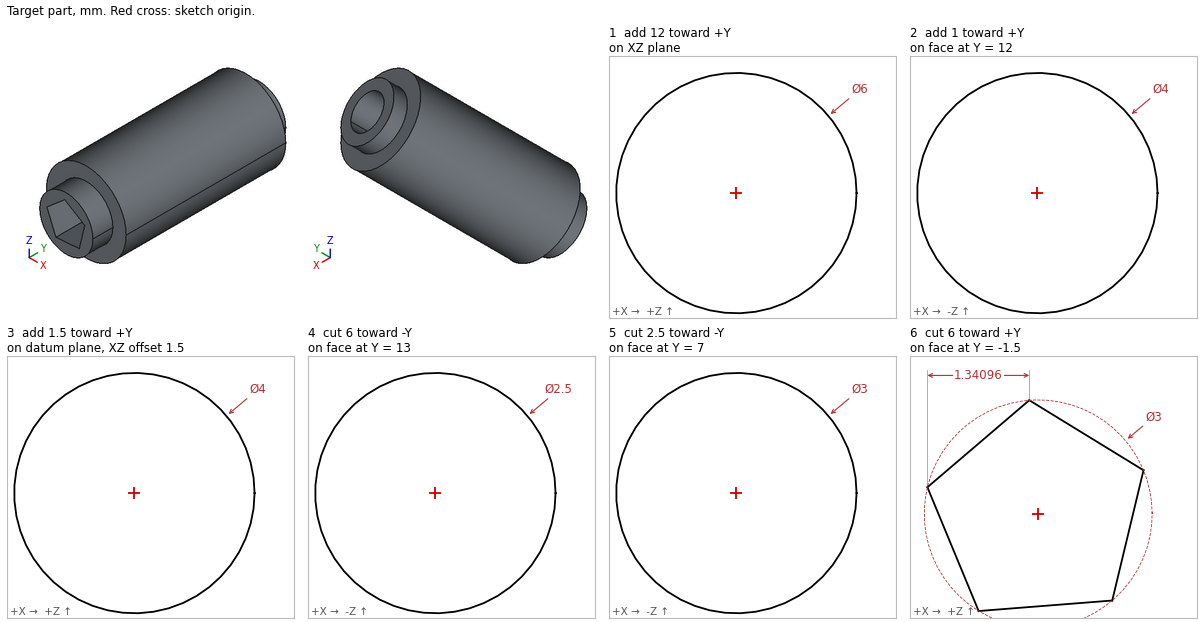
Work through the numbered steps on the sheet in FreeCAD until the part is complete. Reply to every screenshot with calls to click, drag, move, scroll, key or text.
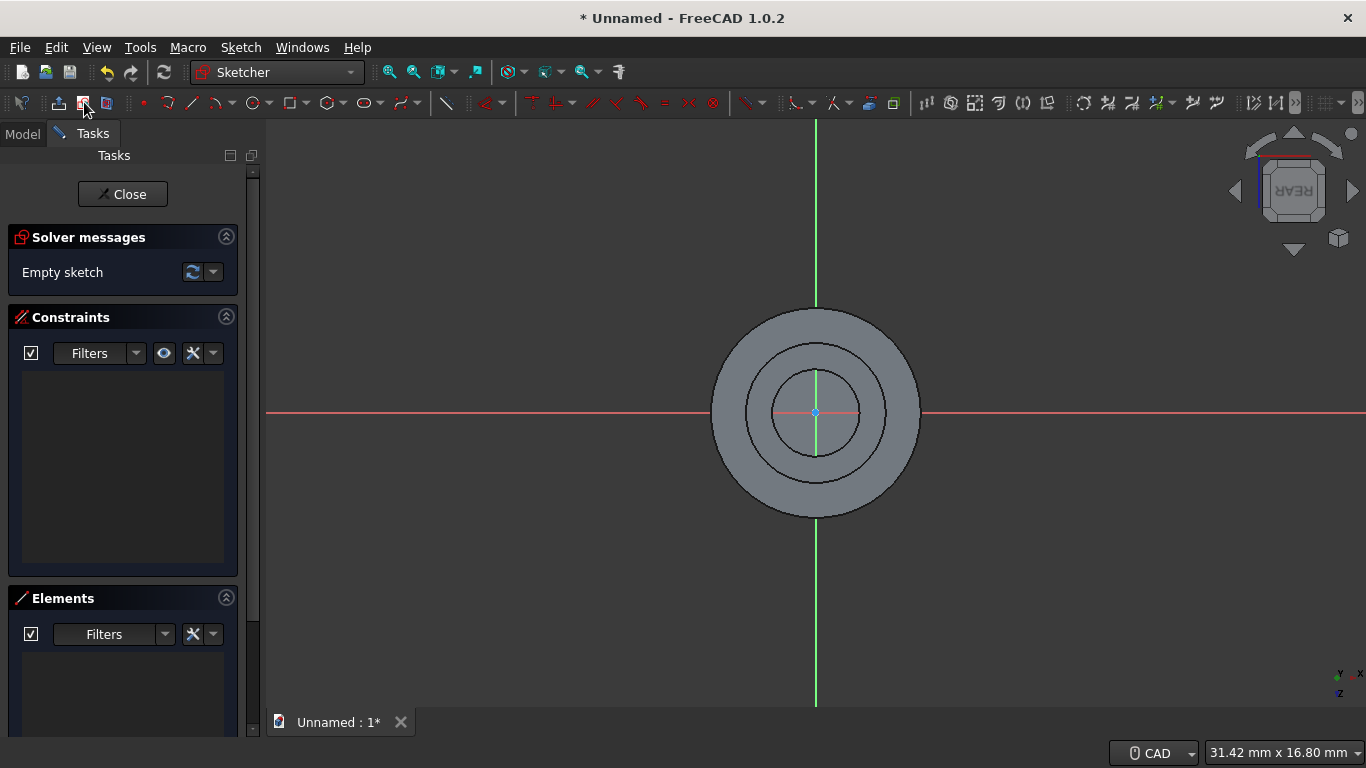
click(108, 104)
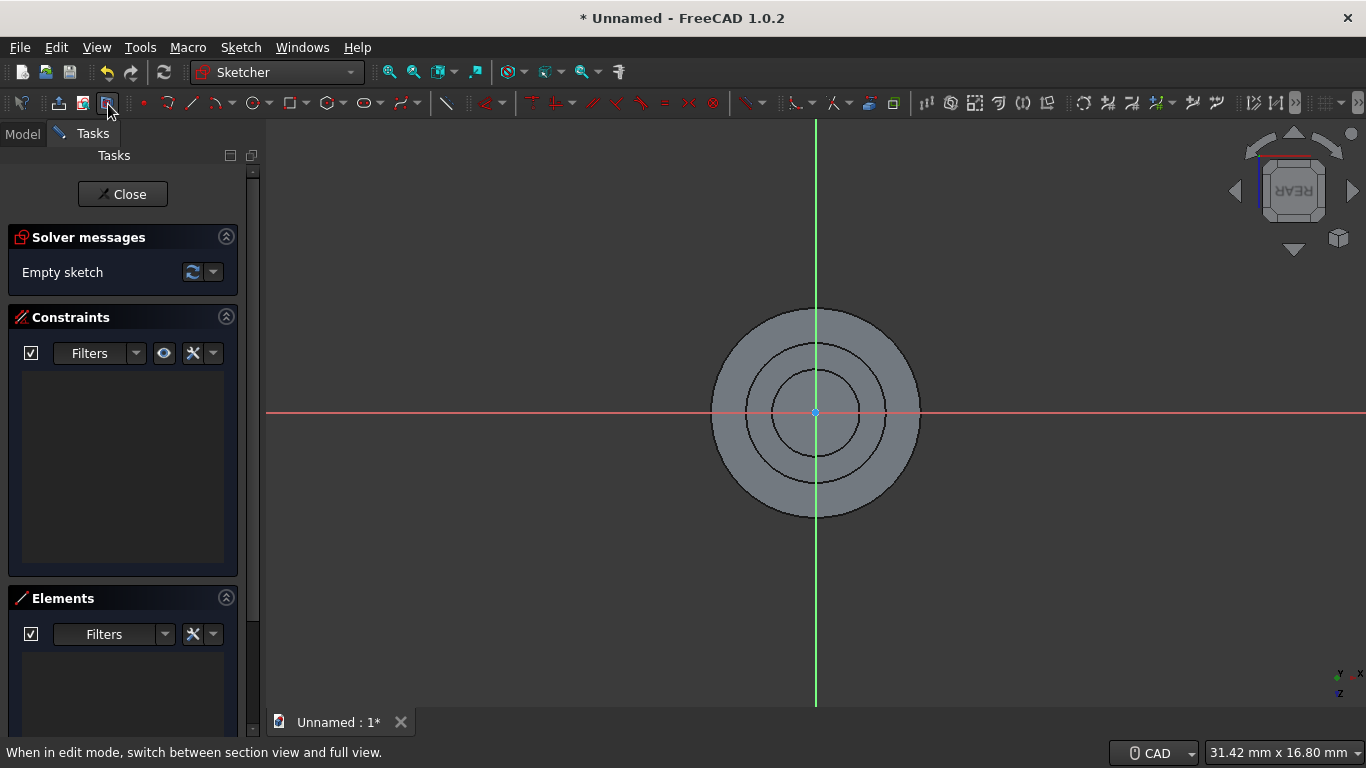
scroll(845, 413, up, 6)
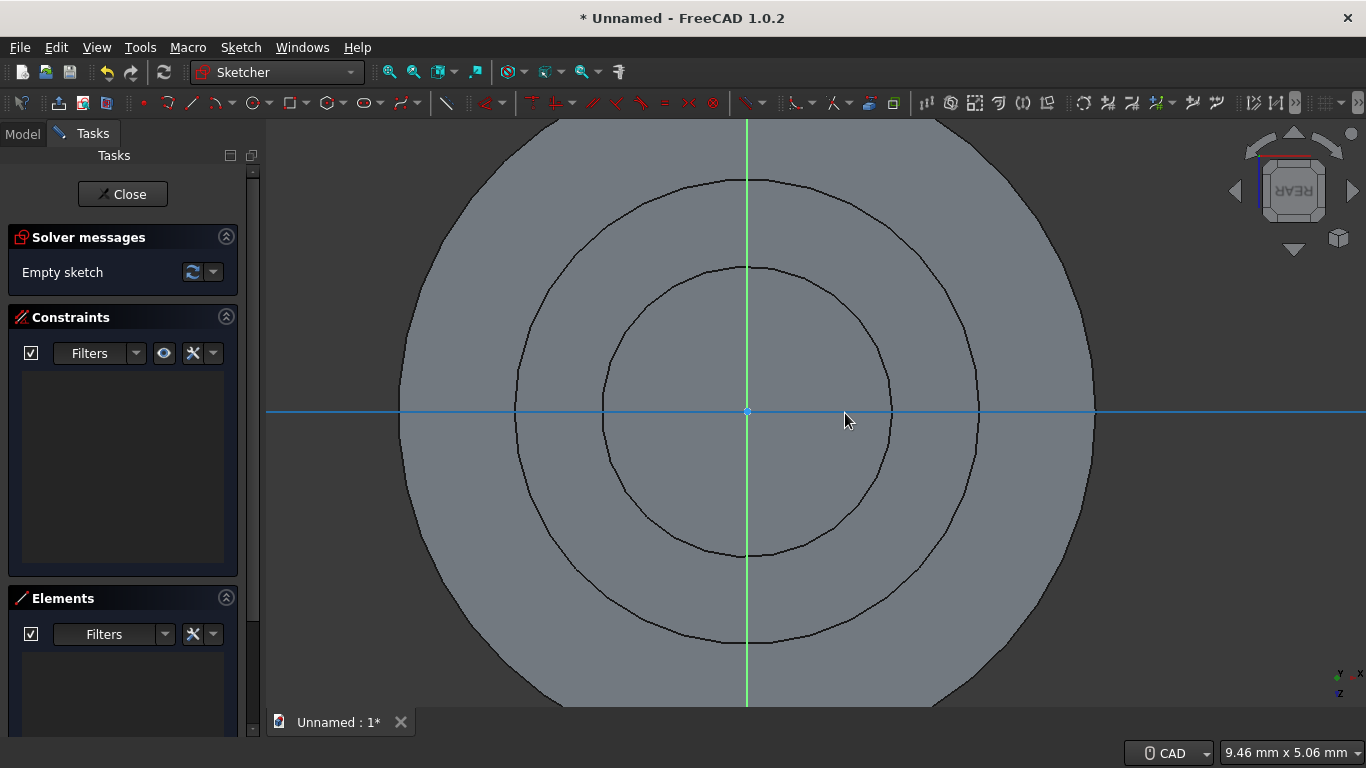
click(254, 104)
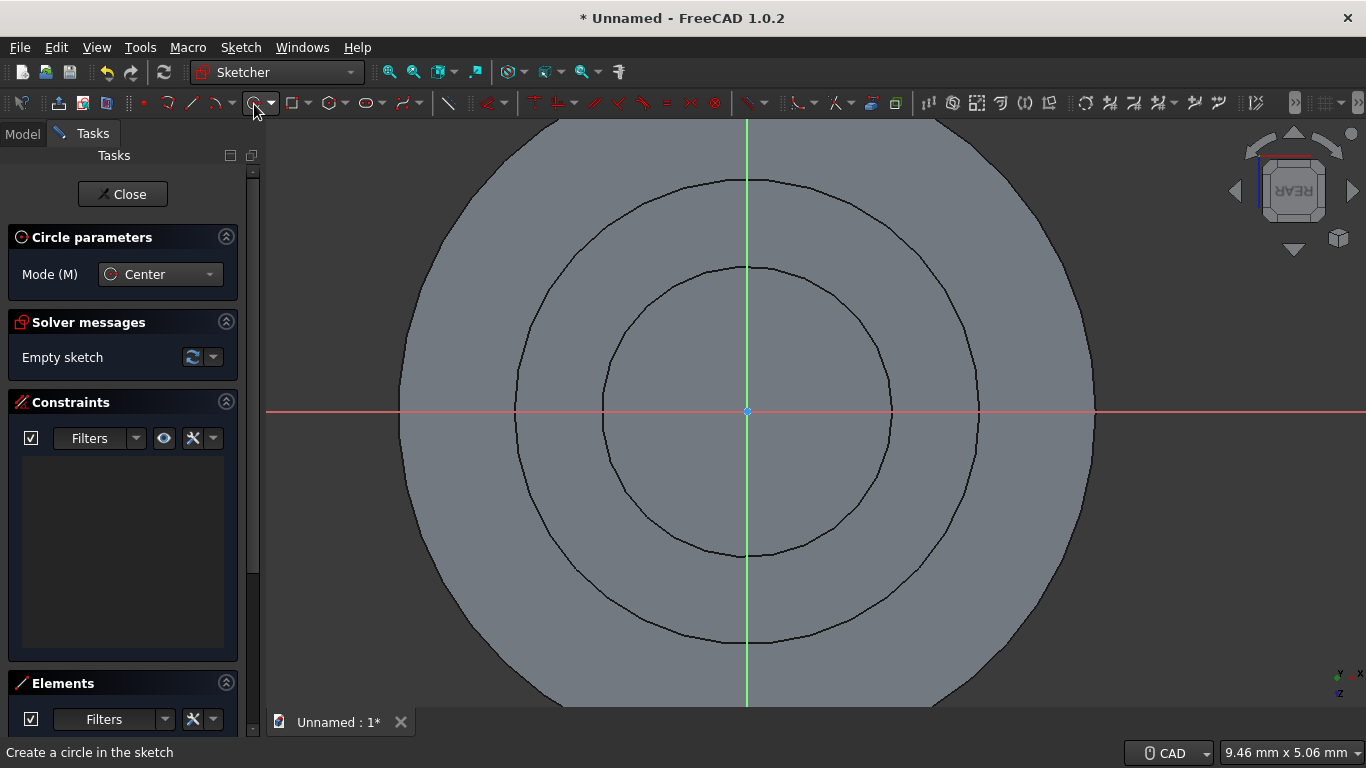
click(747, 412)
move(870, 289)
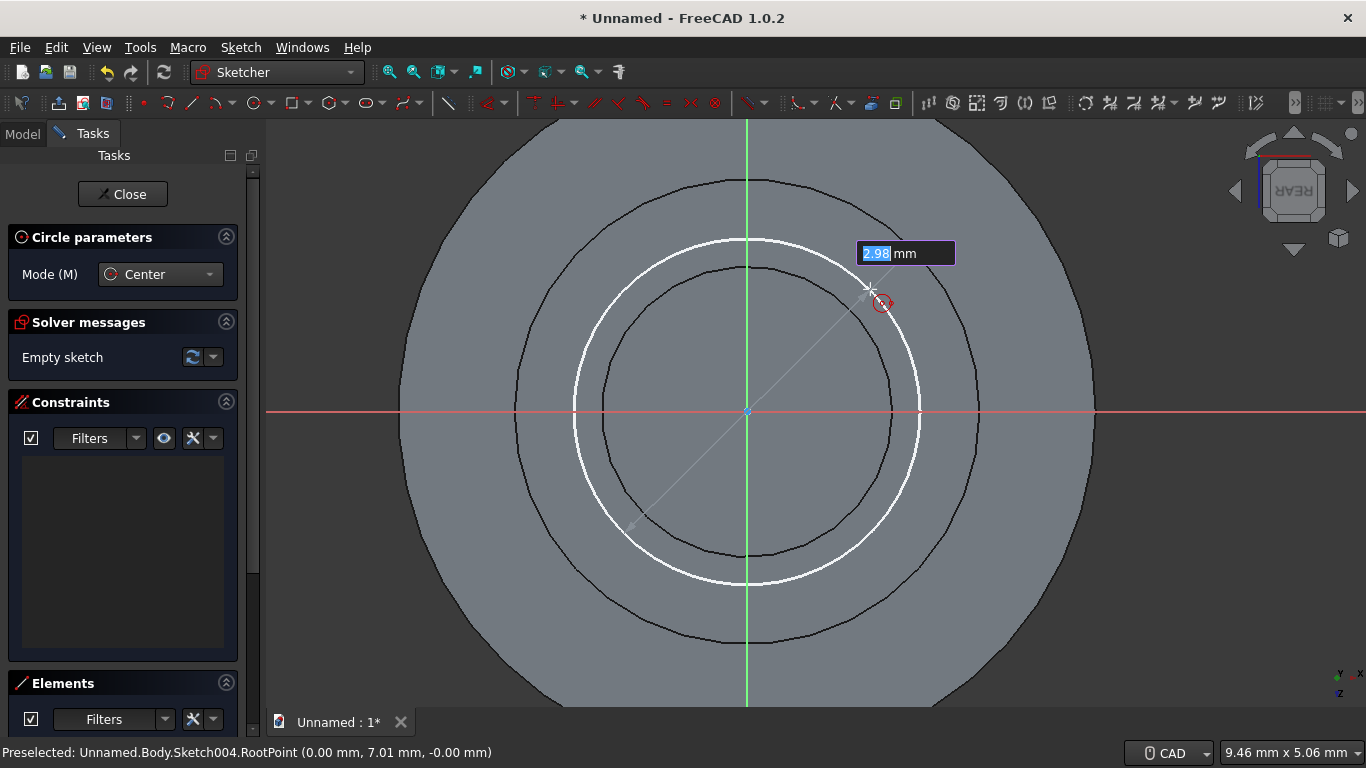
text(3)
key(Return)
key(Escape)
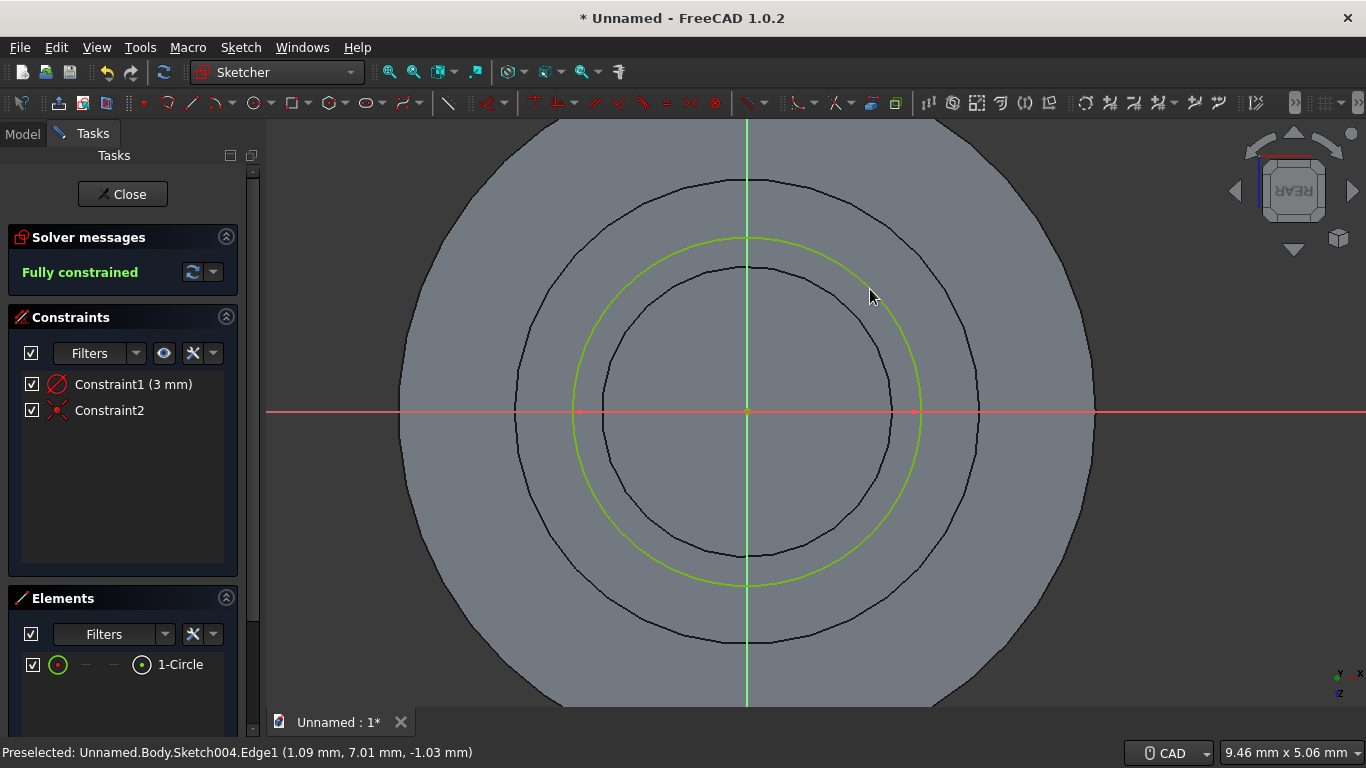
click(123, 194)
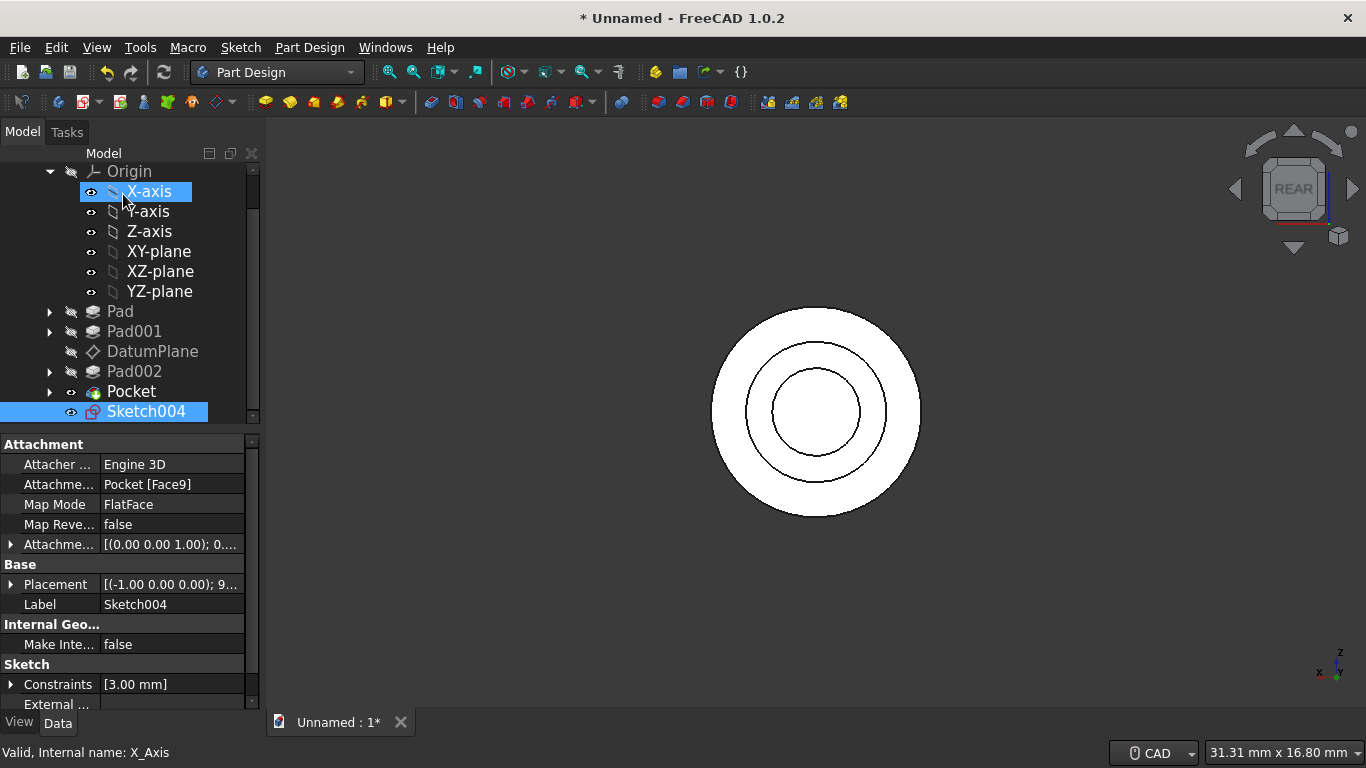
click(432, 102)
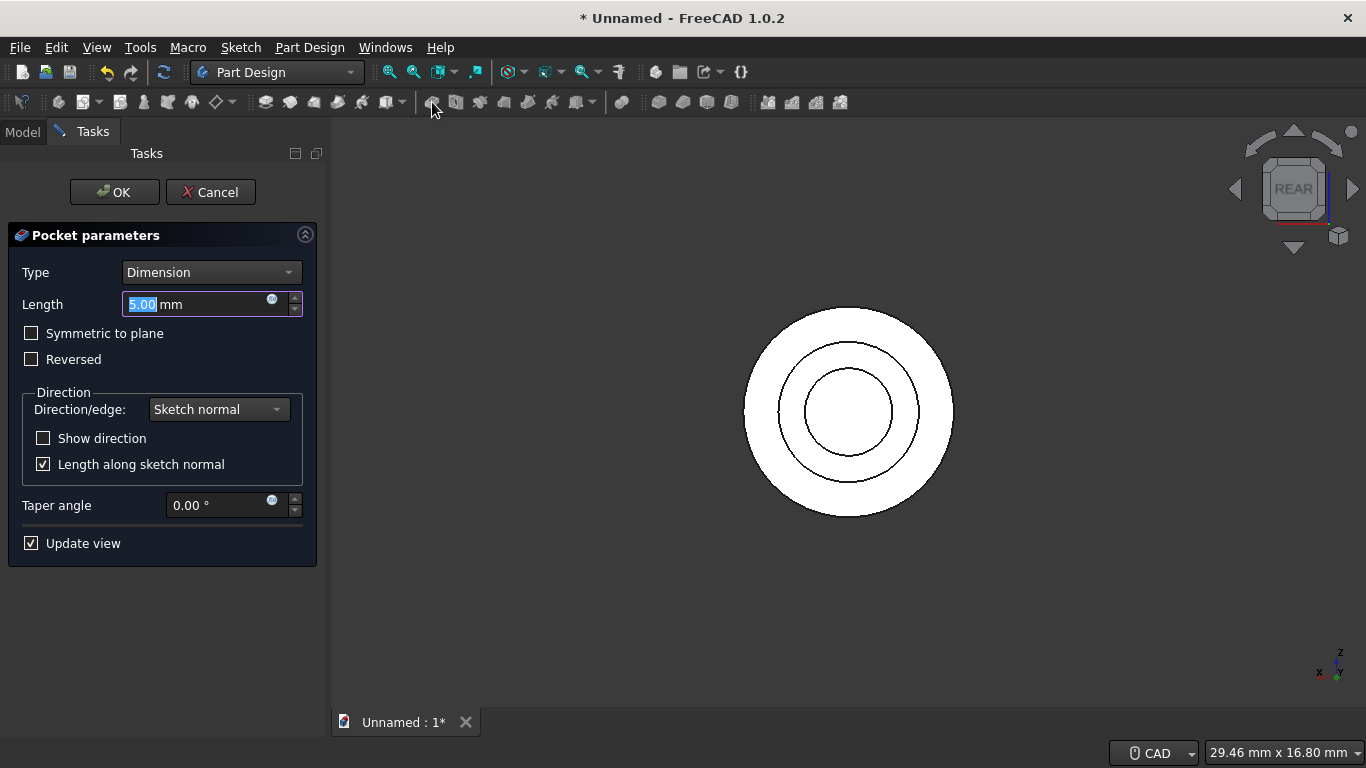
text(2.5)
key(Tab)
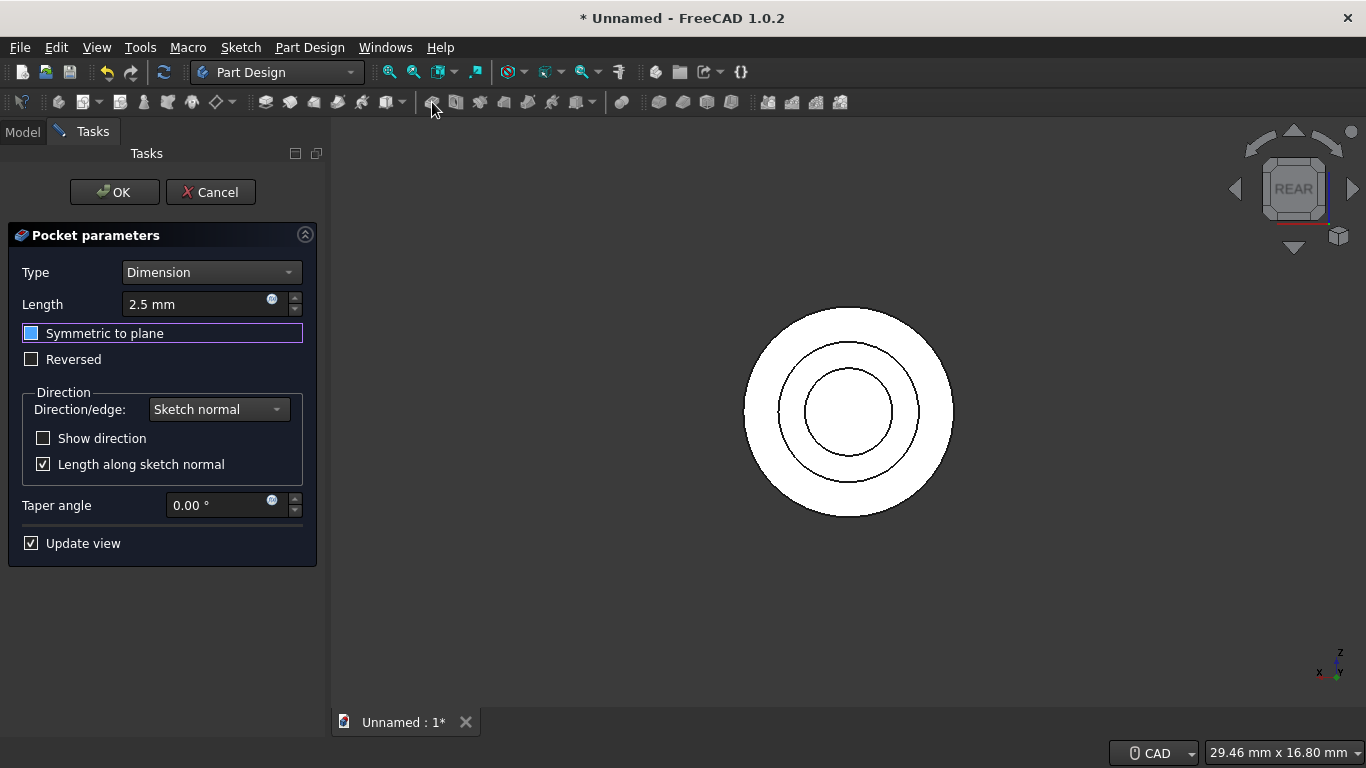
click(115, 192)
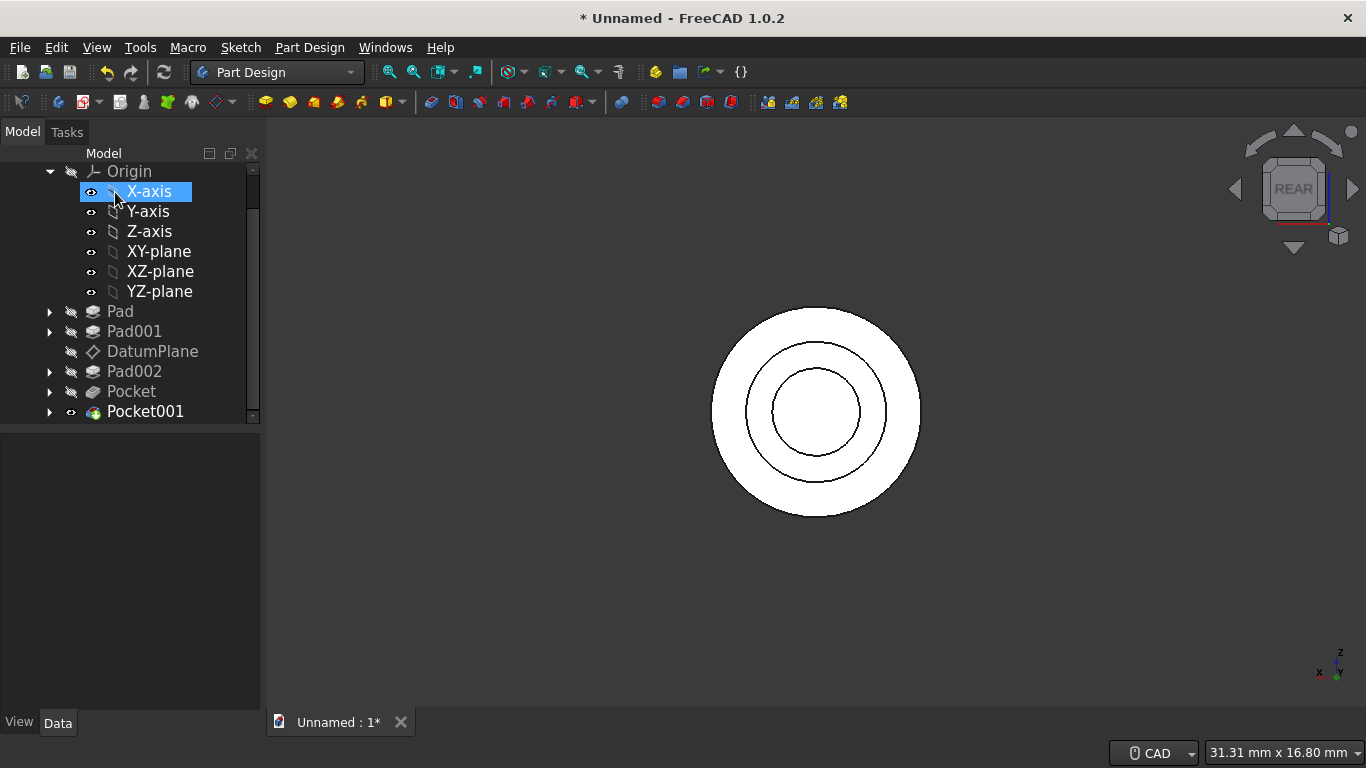
click(390, 72)